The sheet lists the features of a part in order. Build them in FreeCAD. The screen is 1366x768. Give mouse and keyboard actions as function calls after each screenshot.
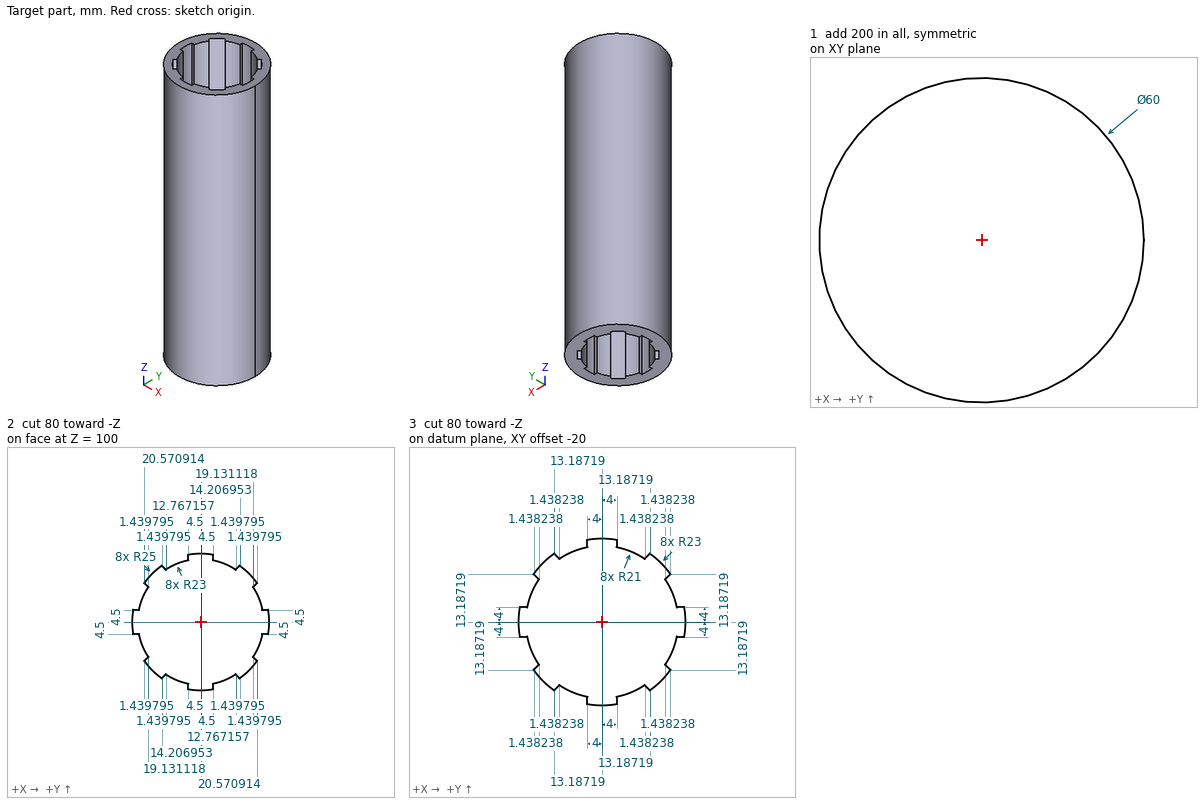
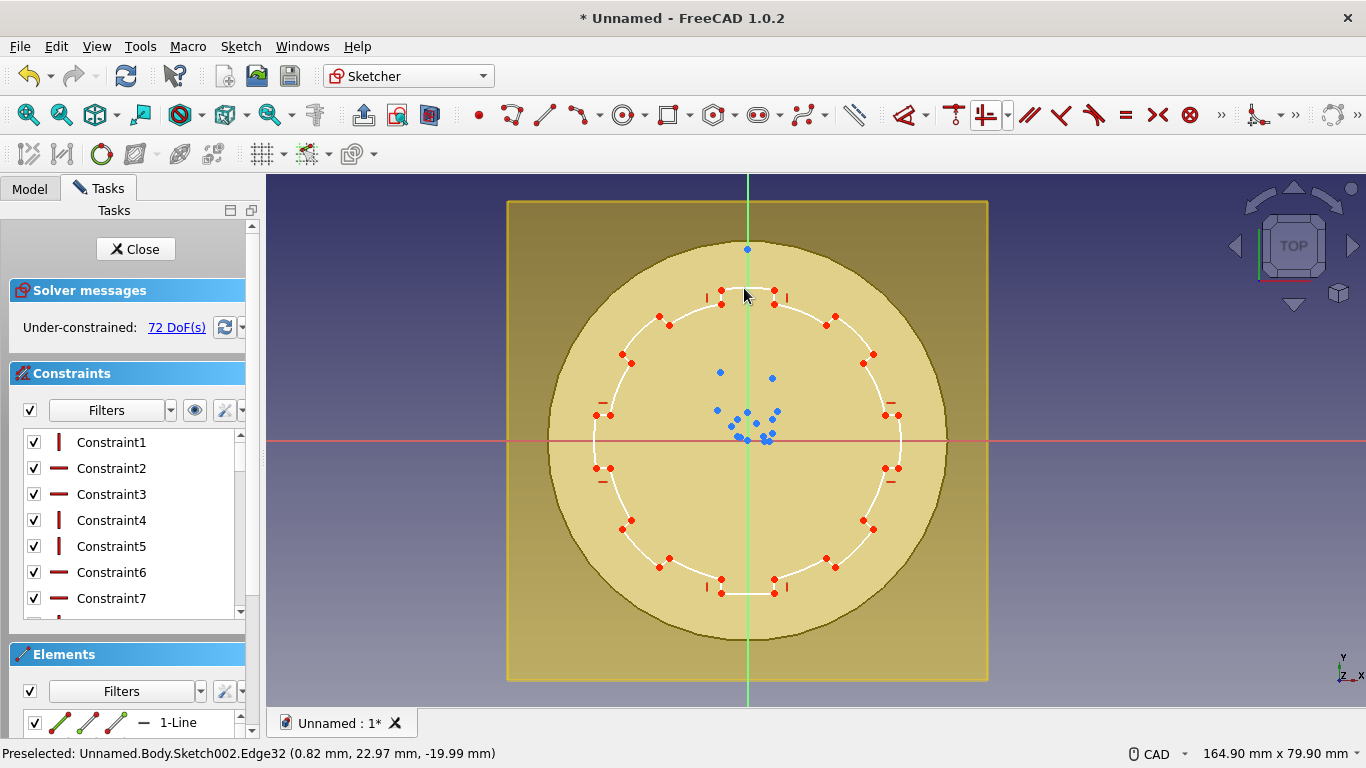
click(791, 308)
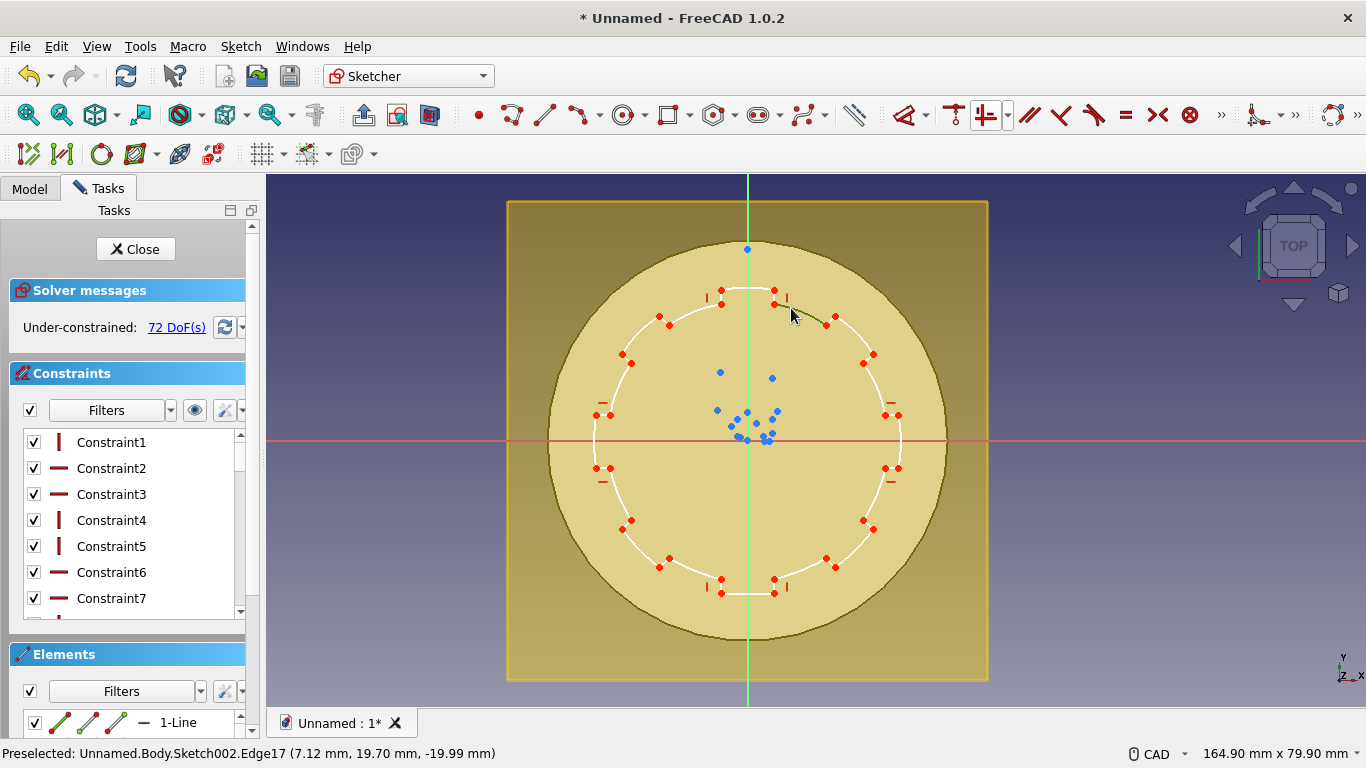
click(864, 341)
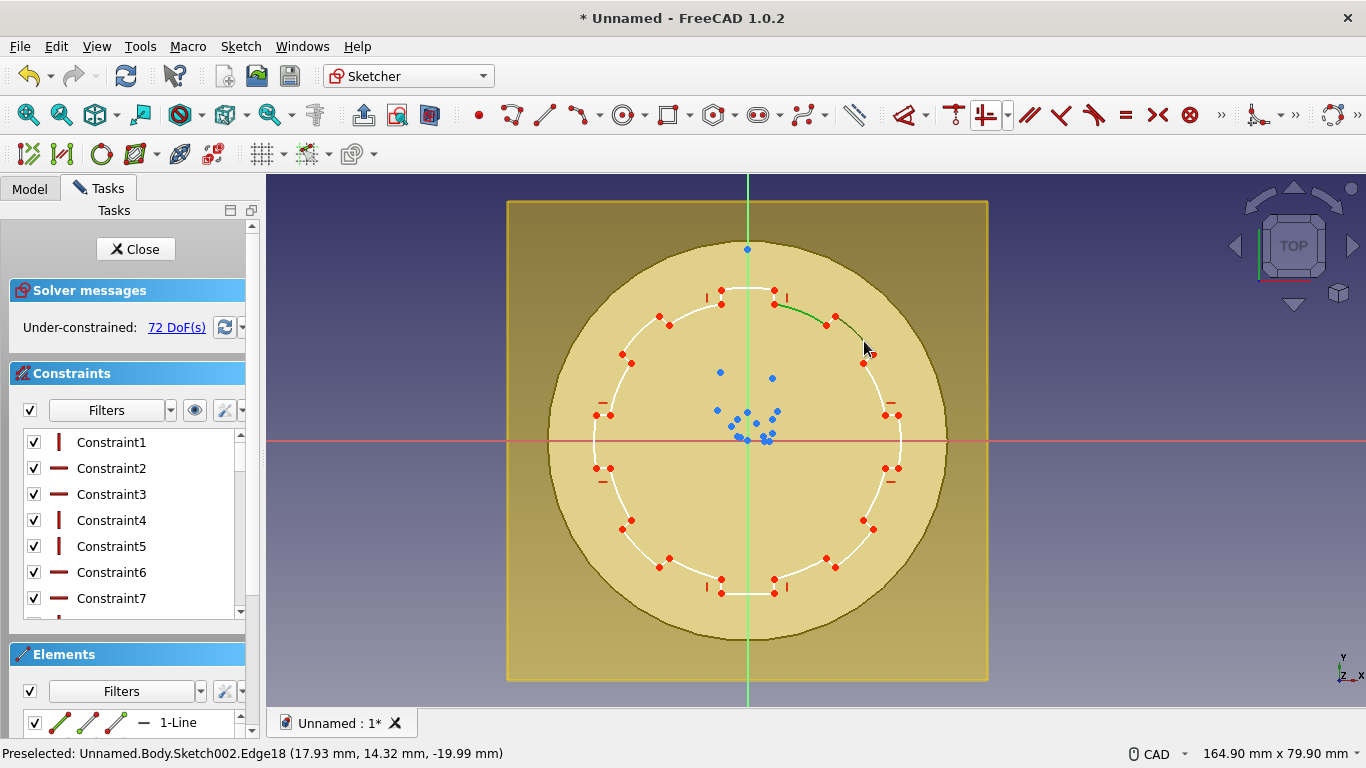
click(954, 116)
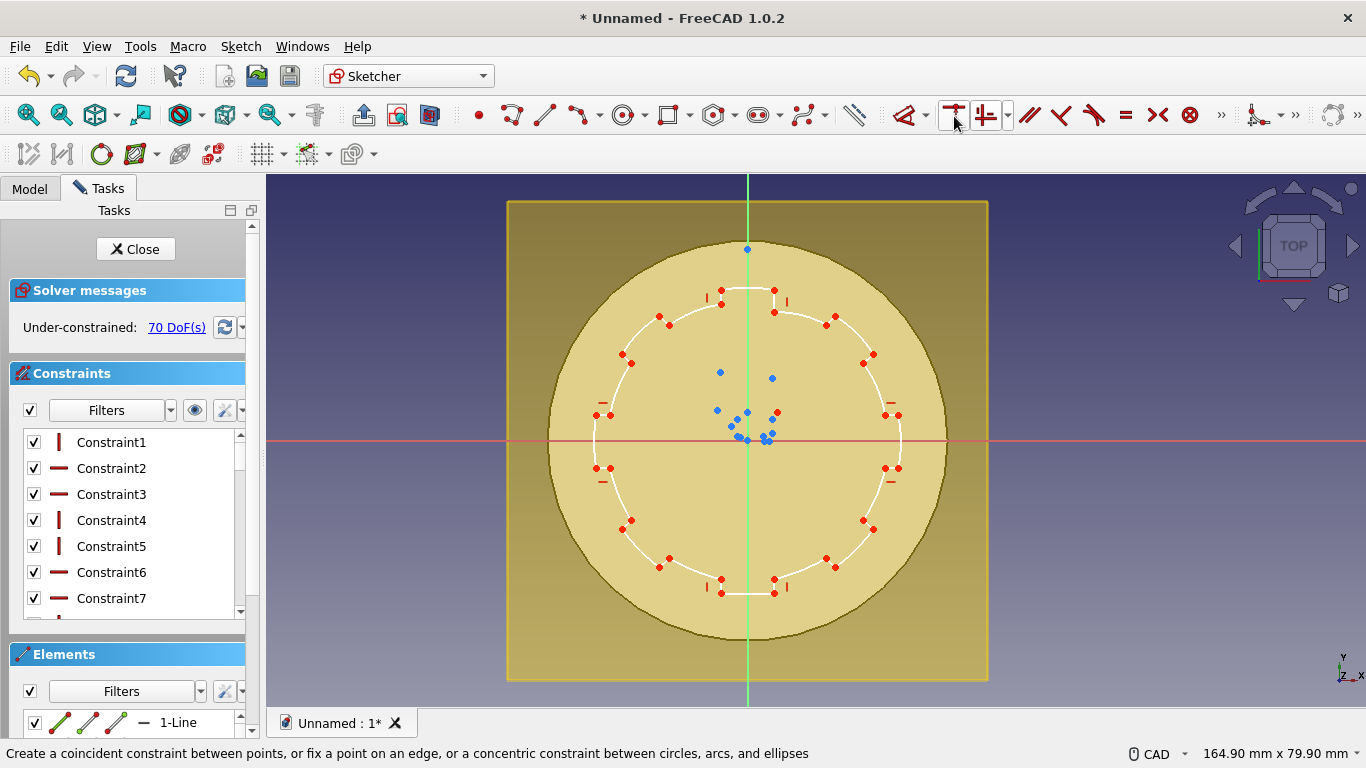
click(812, 318)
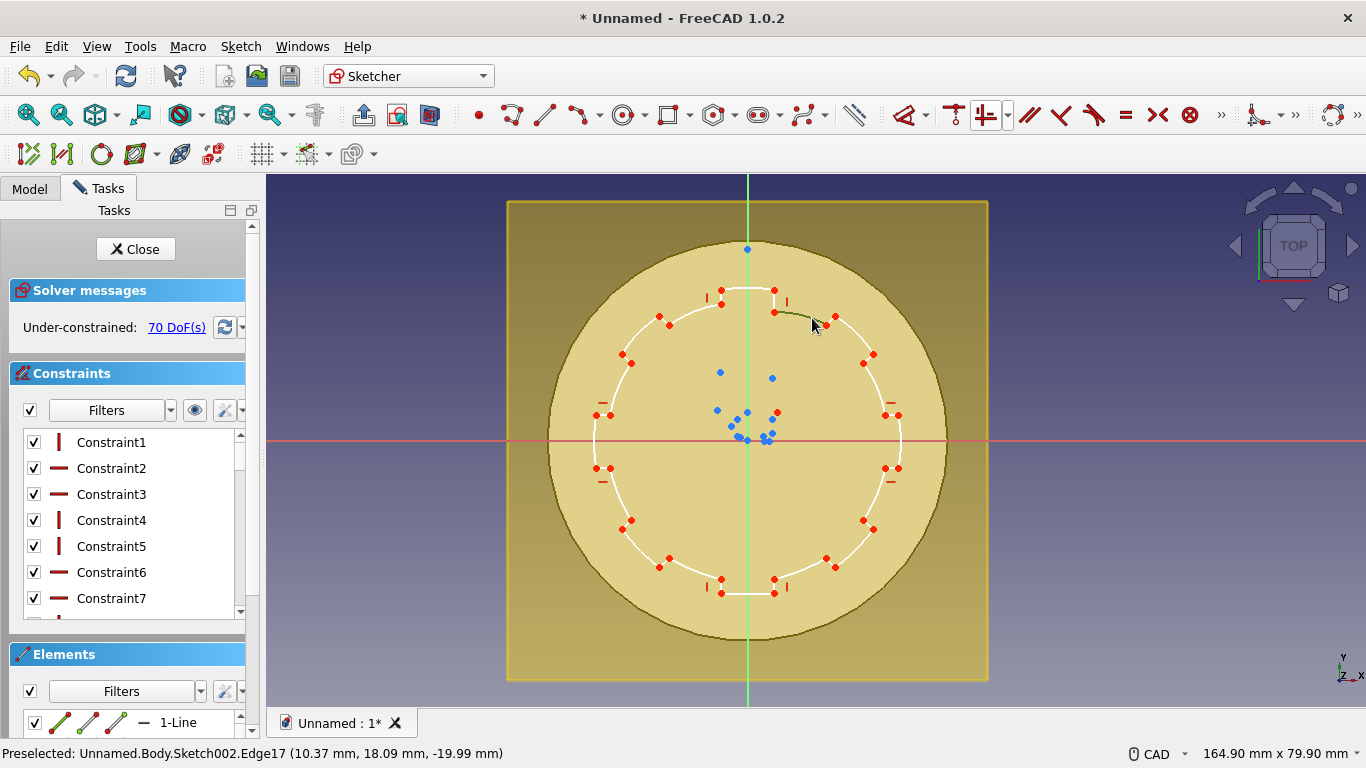
click(881, 399)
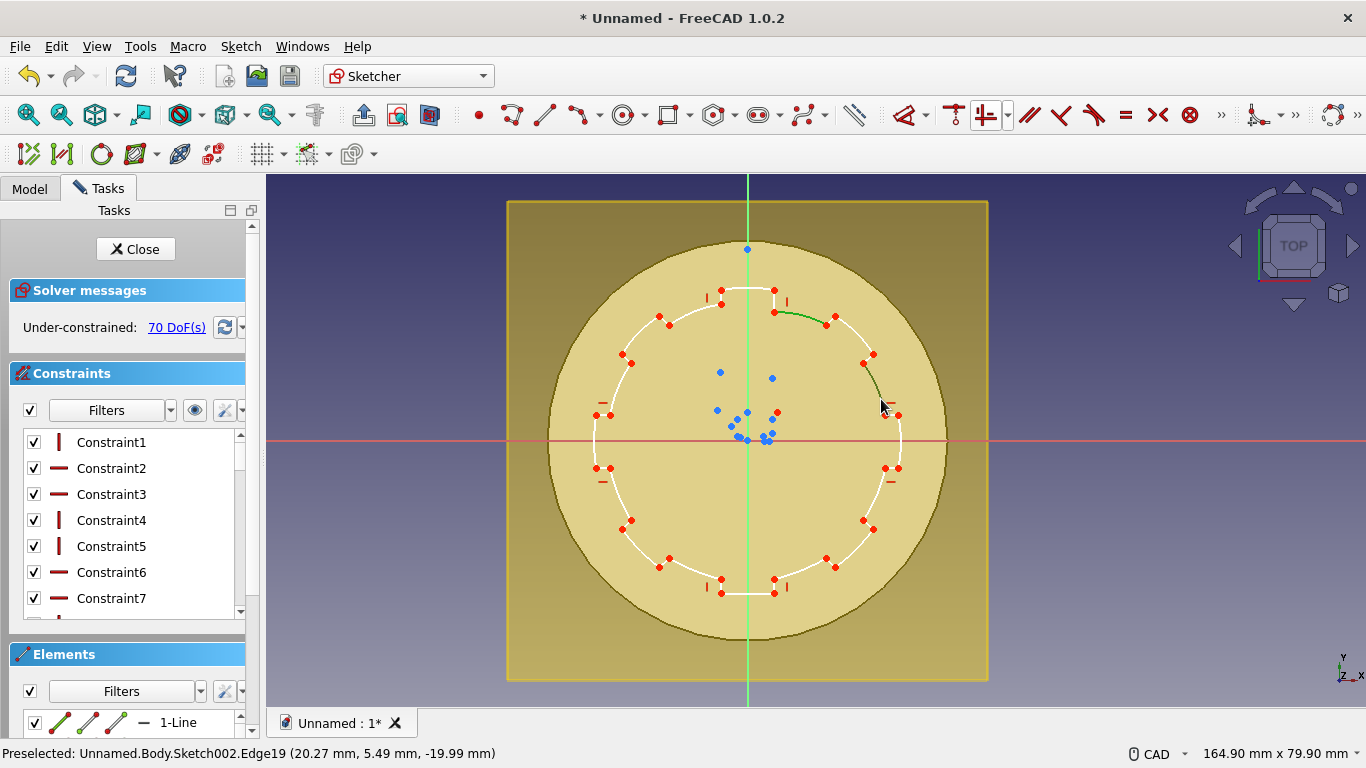
click(954, 116)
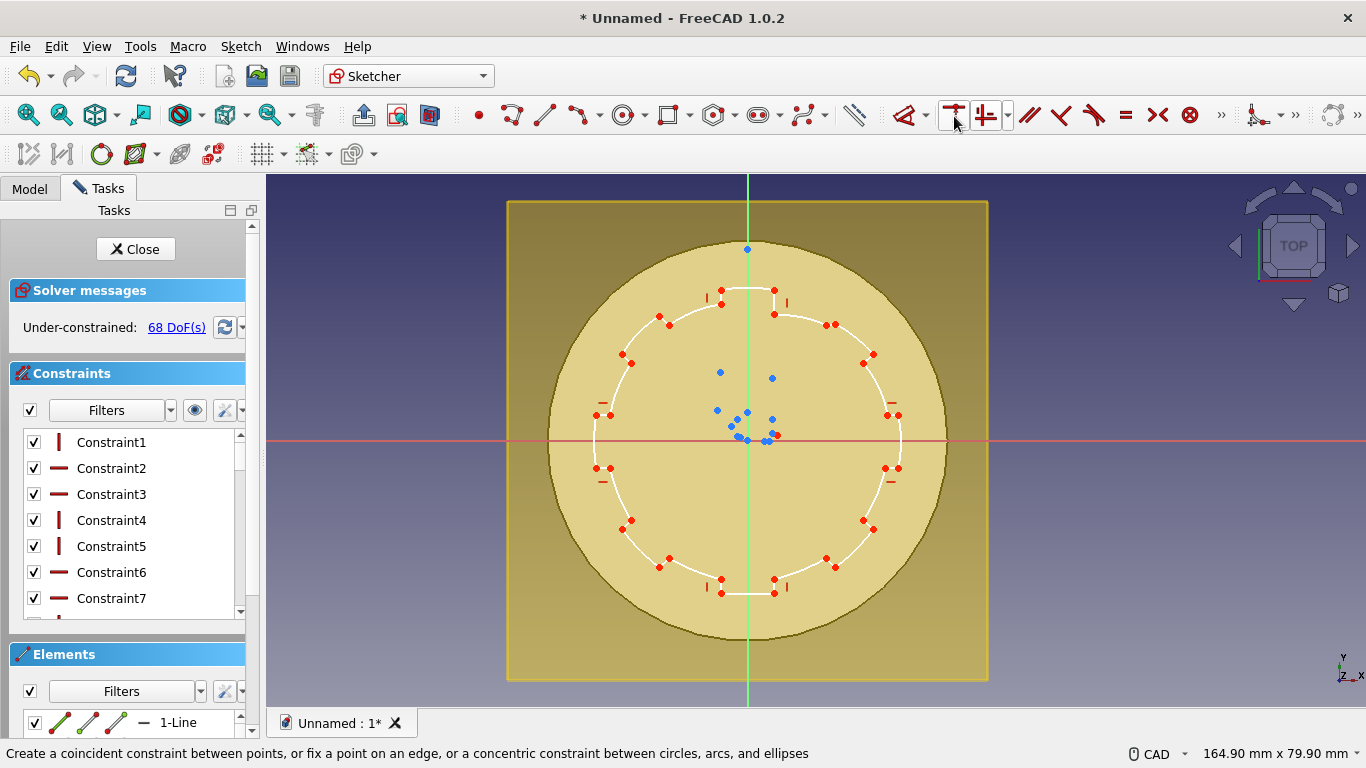
click(811, 320)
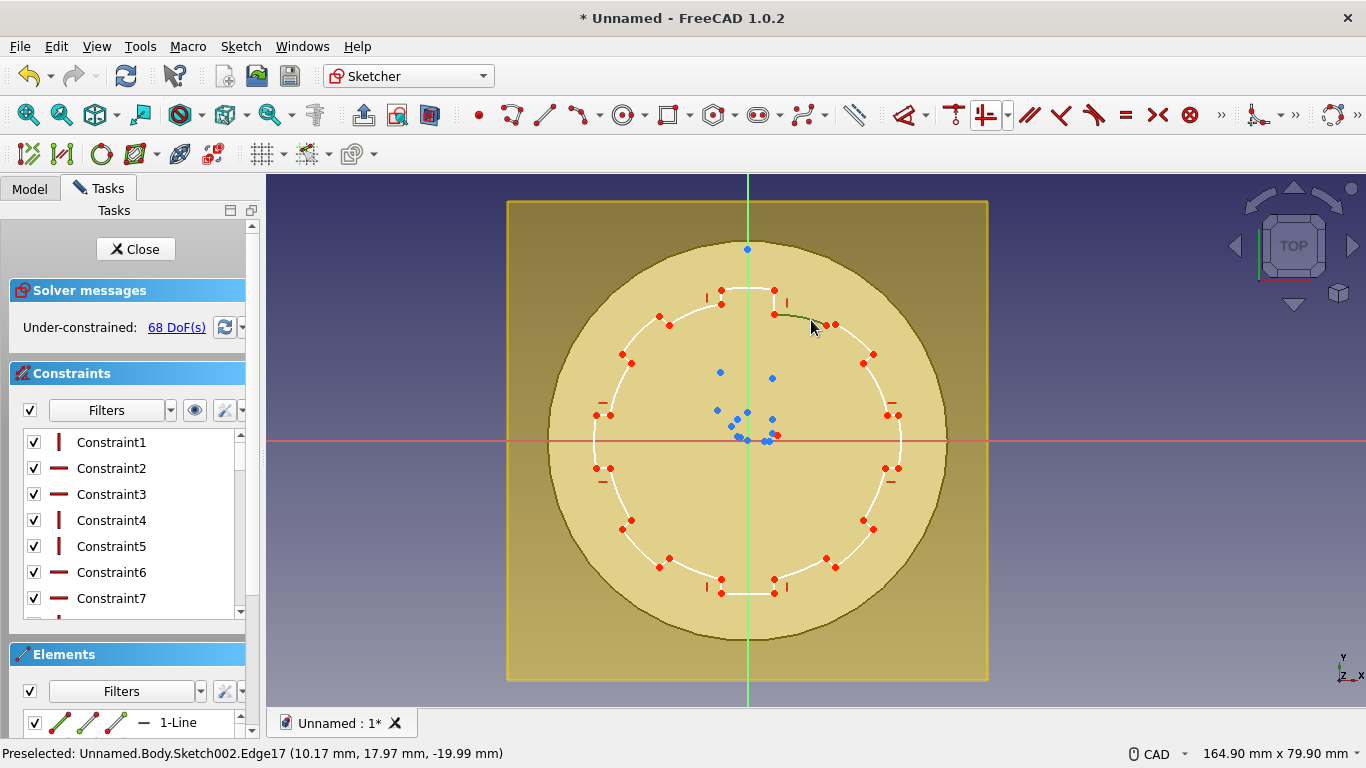
click(900, 453)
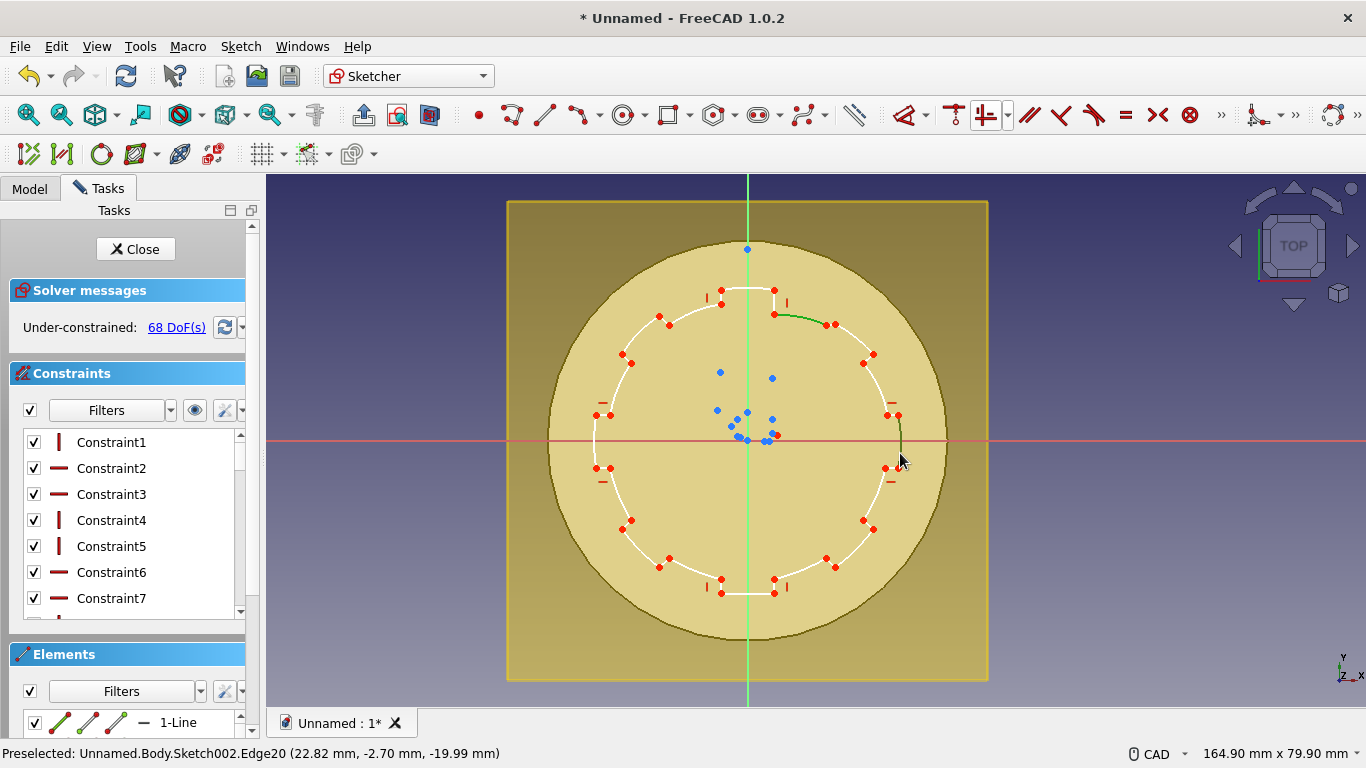
click(954, 116)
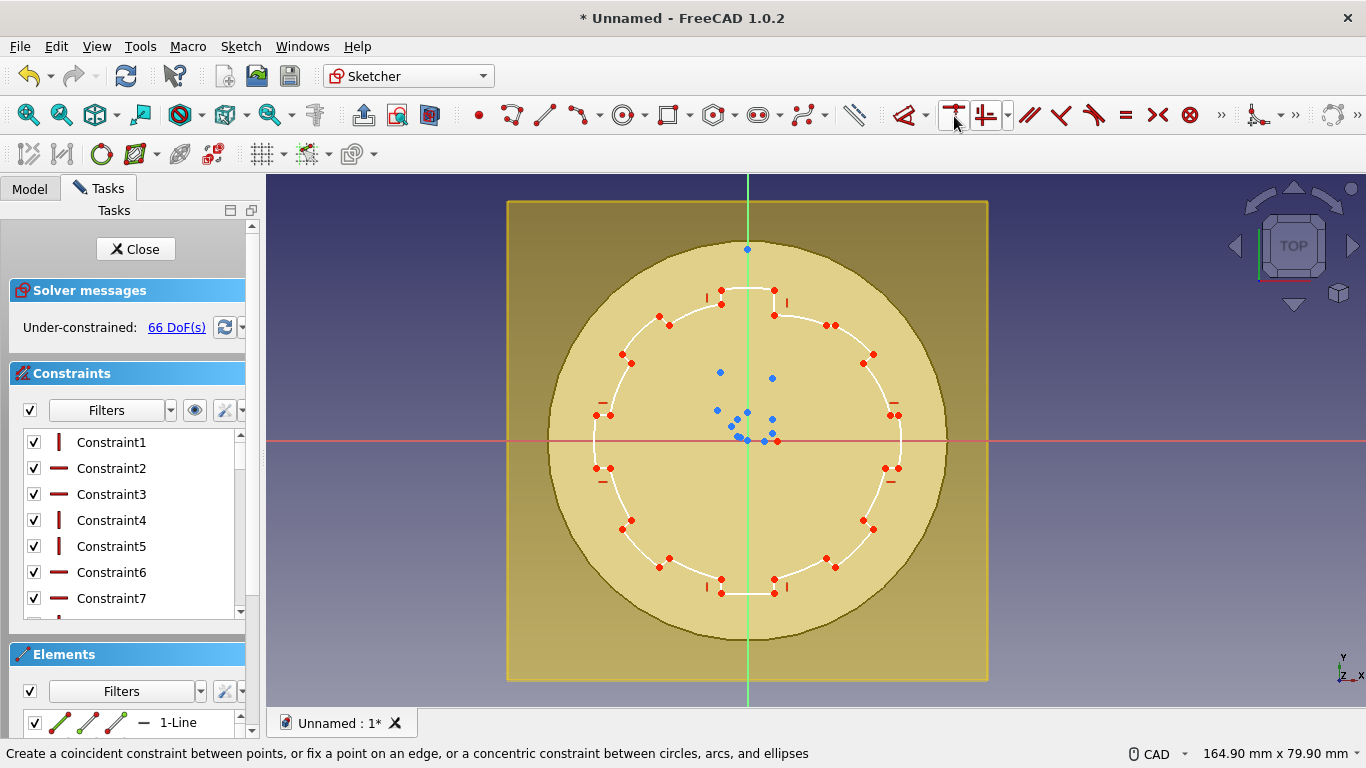
click(811, 320)